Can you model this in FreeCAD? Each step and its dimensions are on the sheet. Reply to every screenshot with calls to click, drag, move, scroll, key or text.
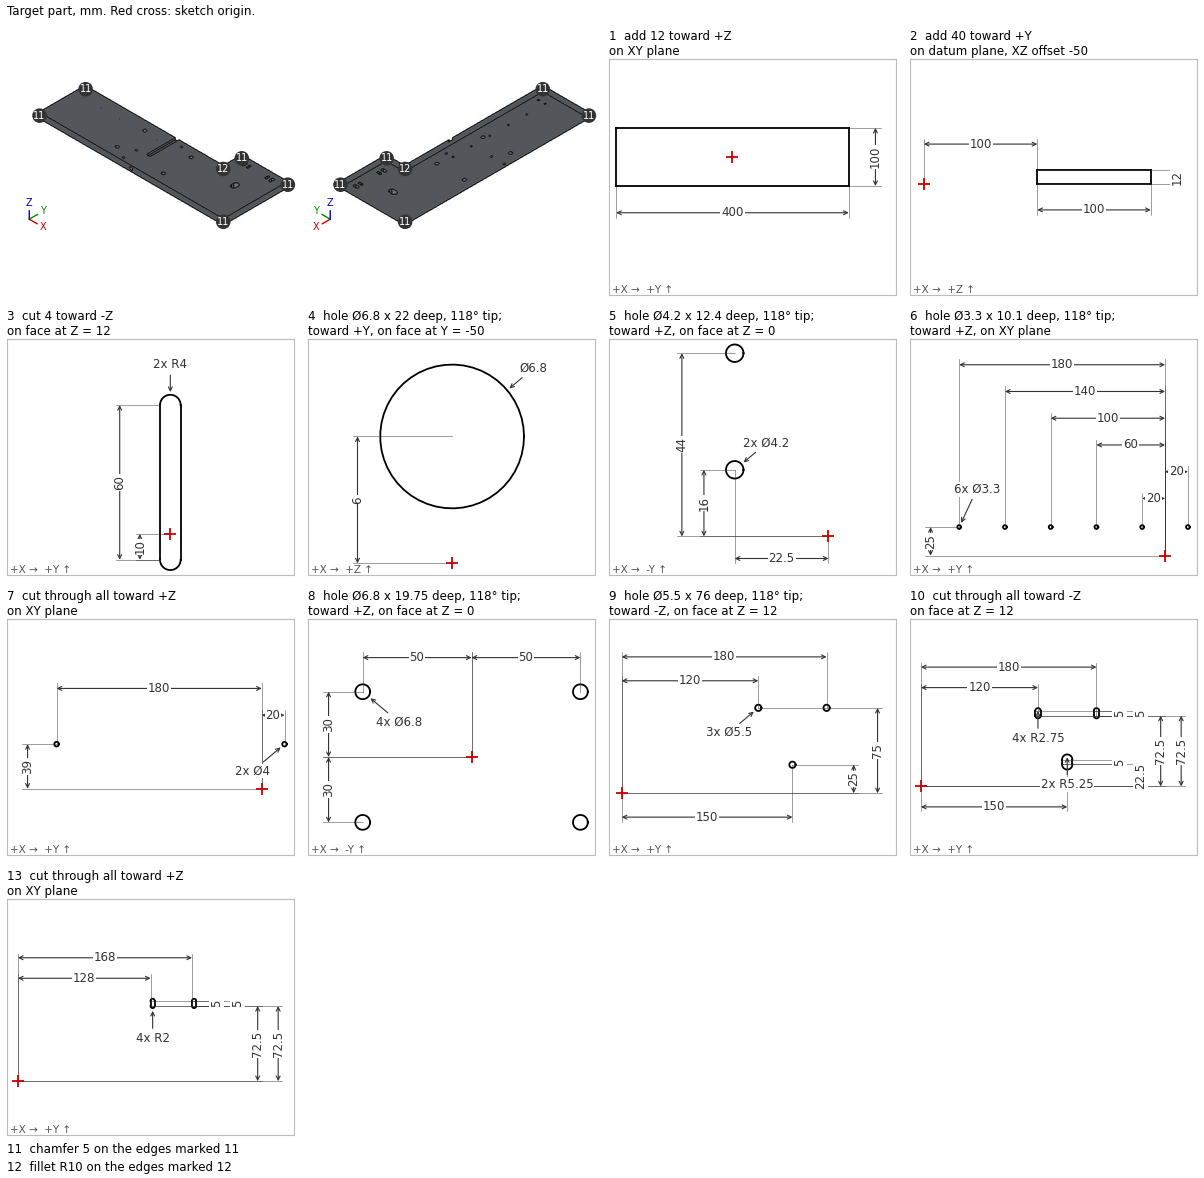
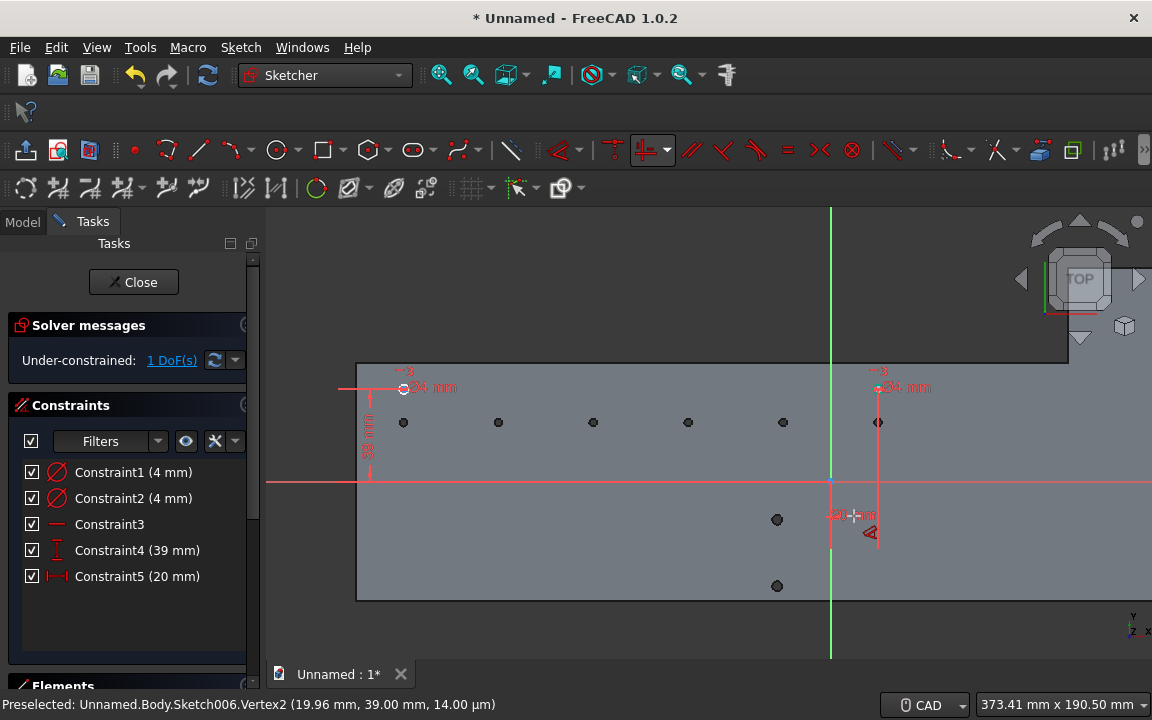
click(404, 389)
click(617, 516)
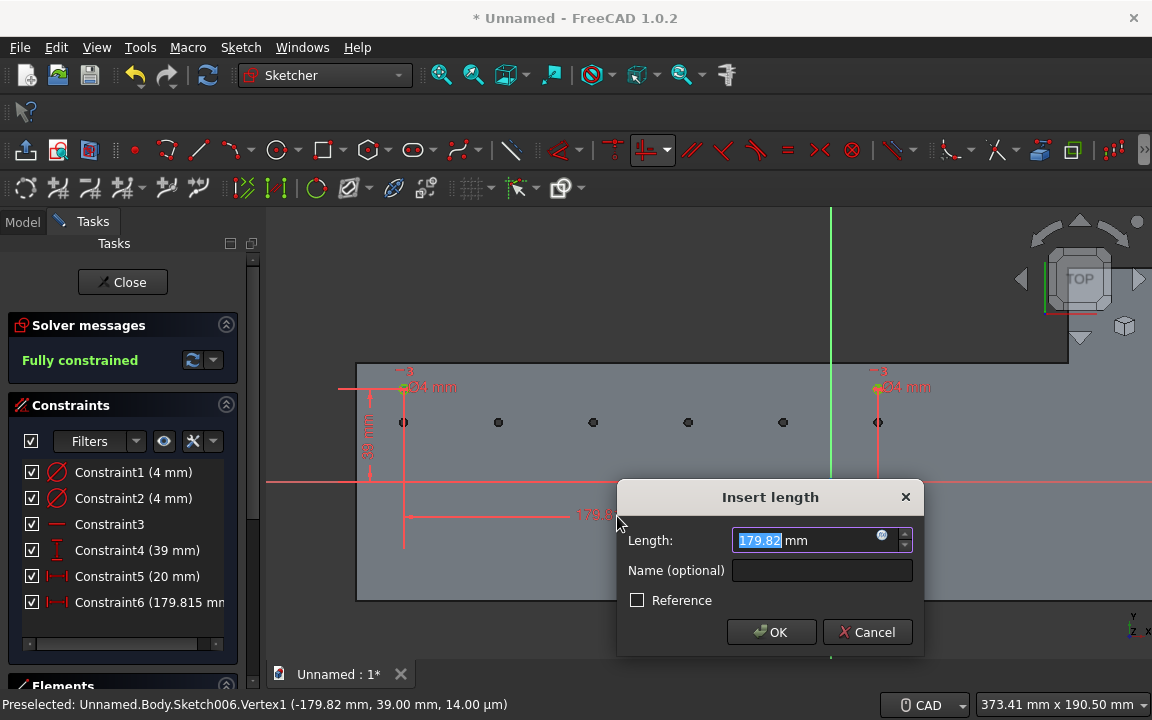
text(180)
key(Return)
key(Escape)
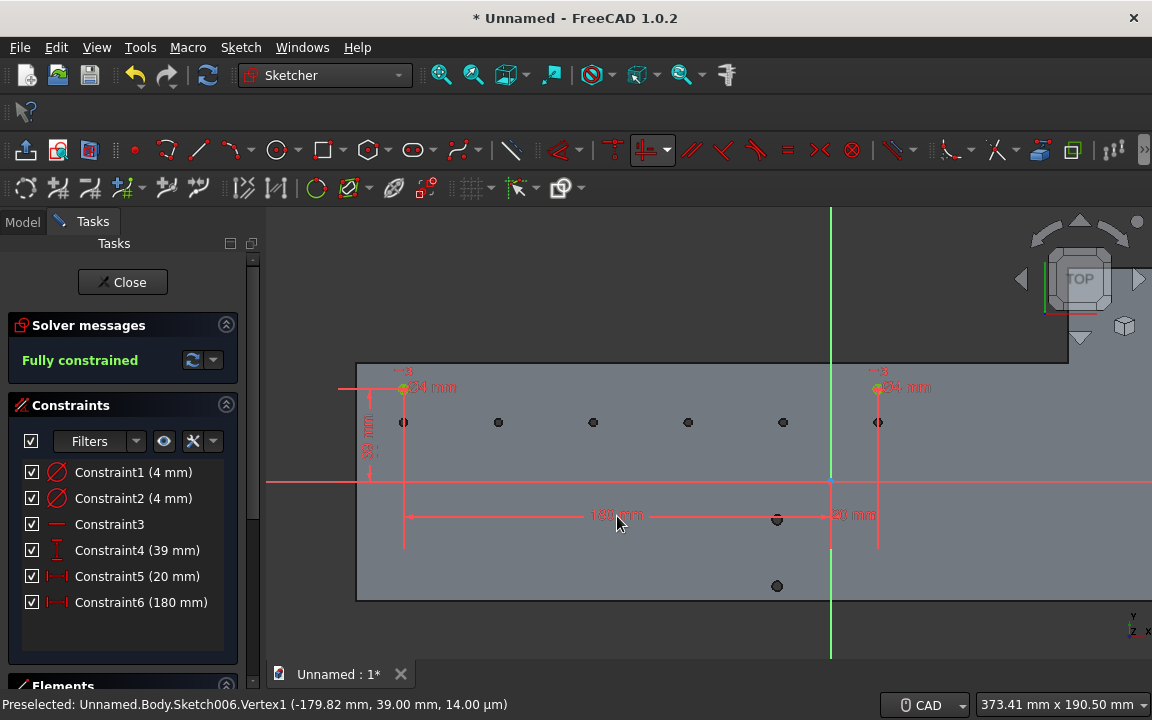
click(123, 282)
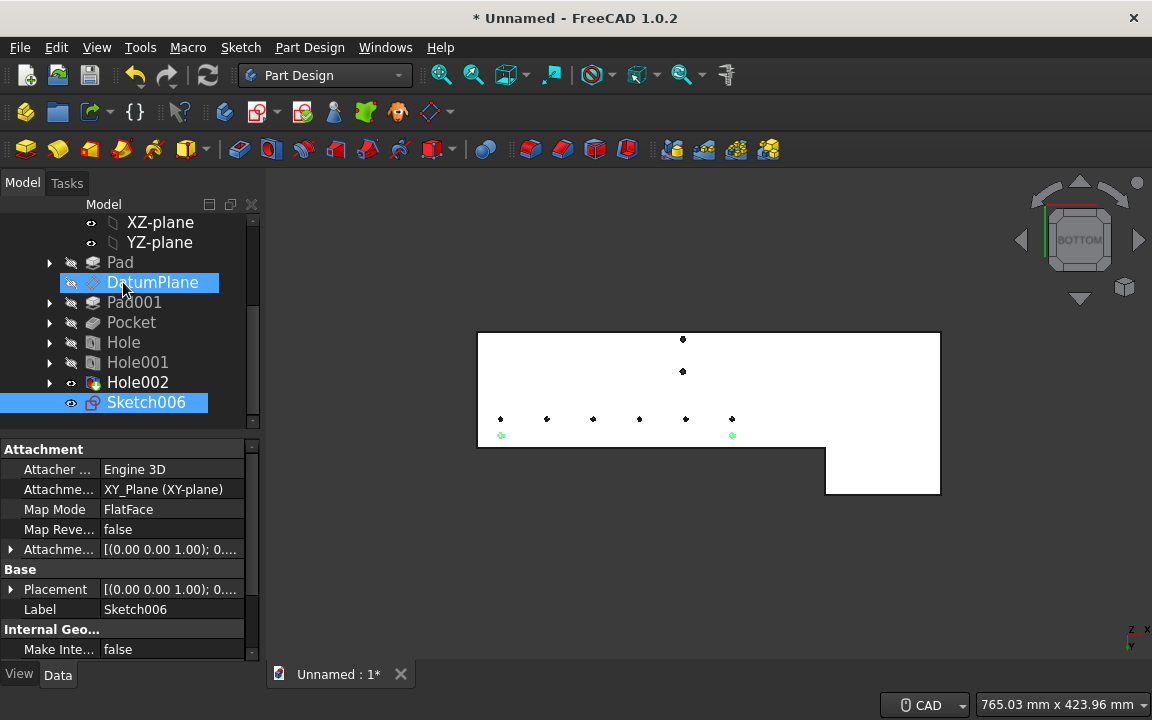
click(240, 150)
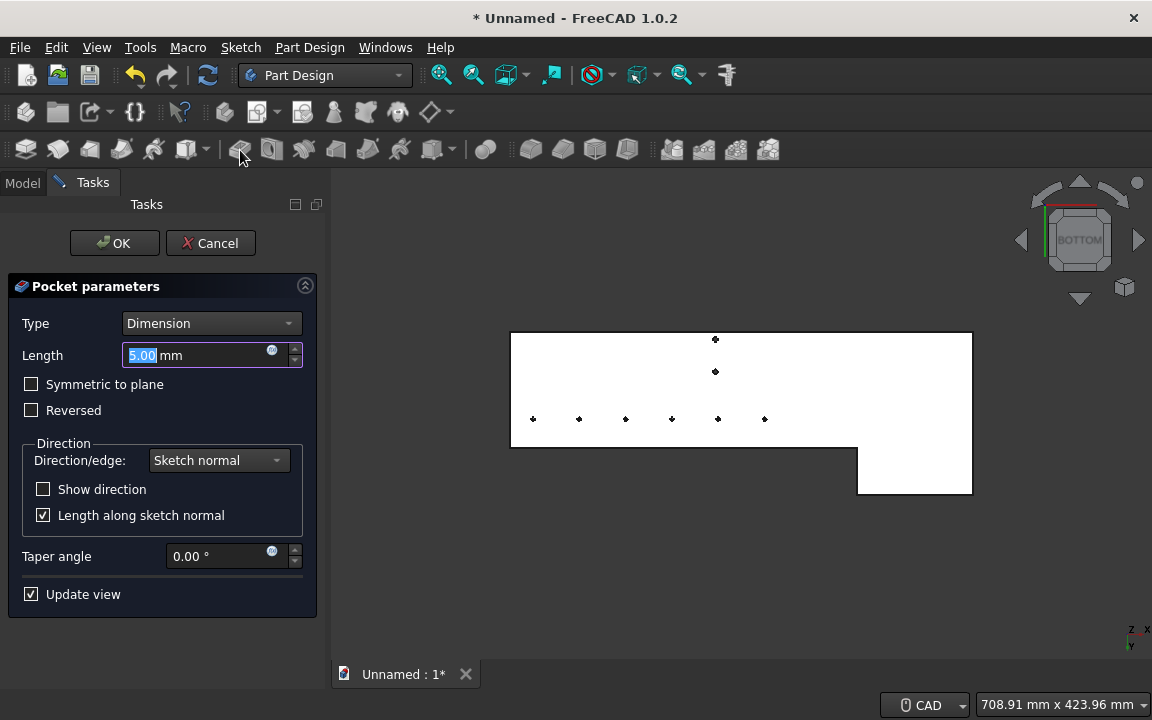
click(212, 324)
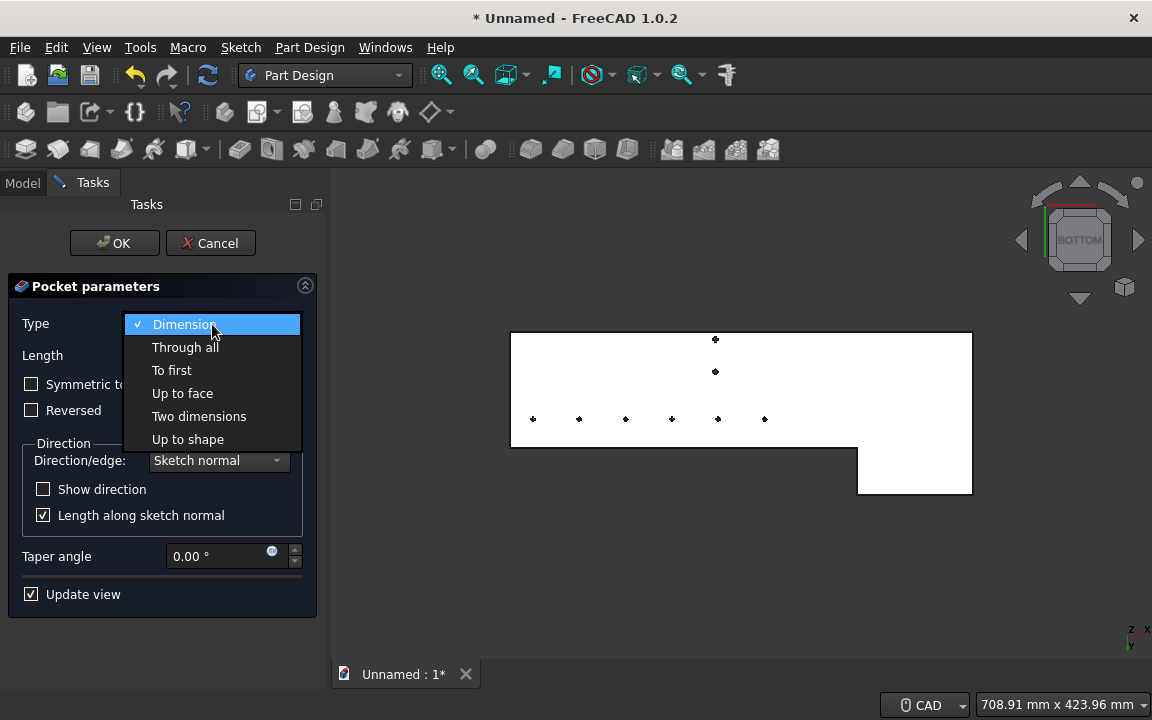
click(212, 348)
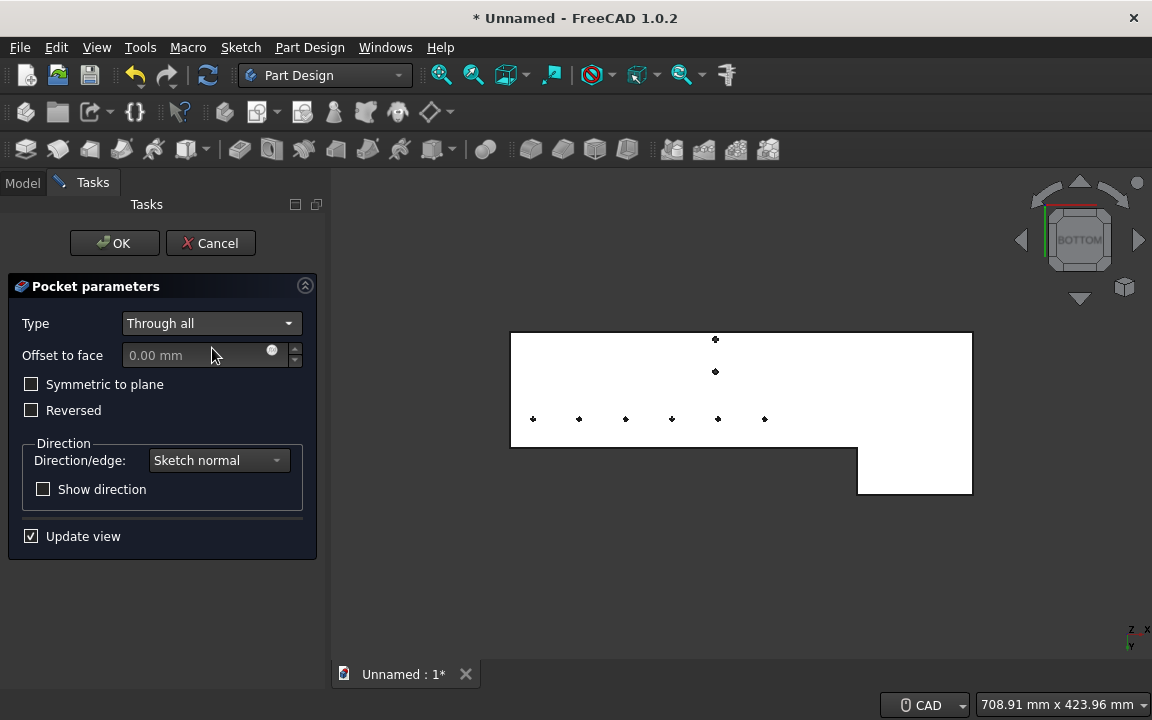
click(30, 410)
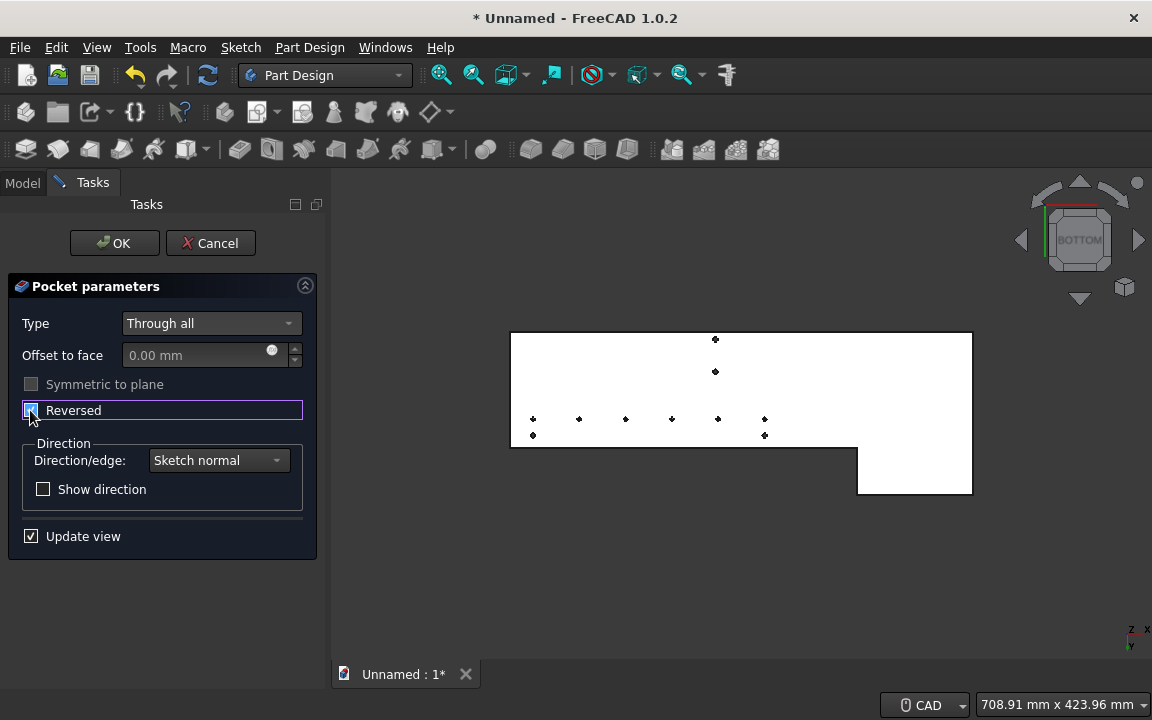
click(115, 243)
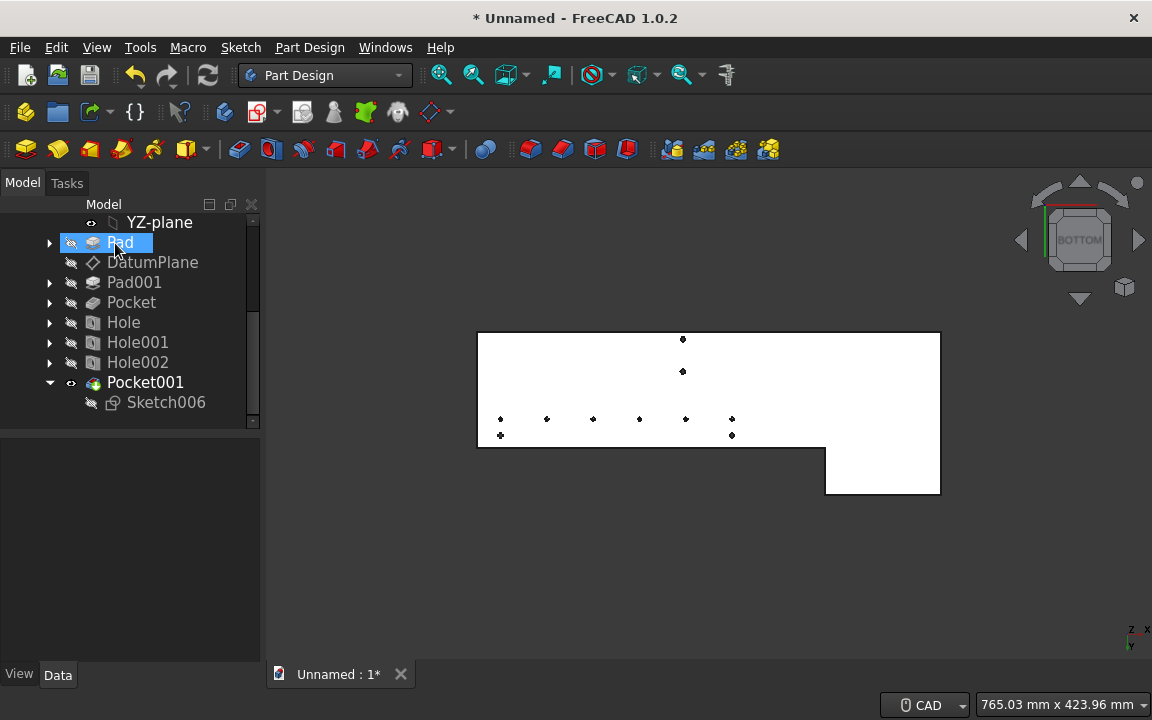
click(841, 389)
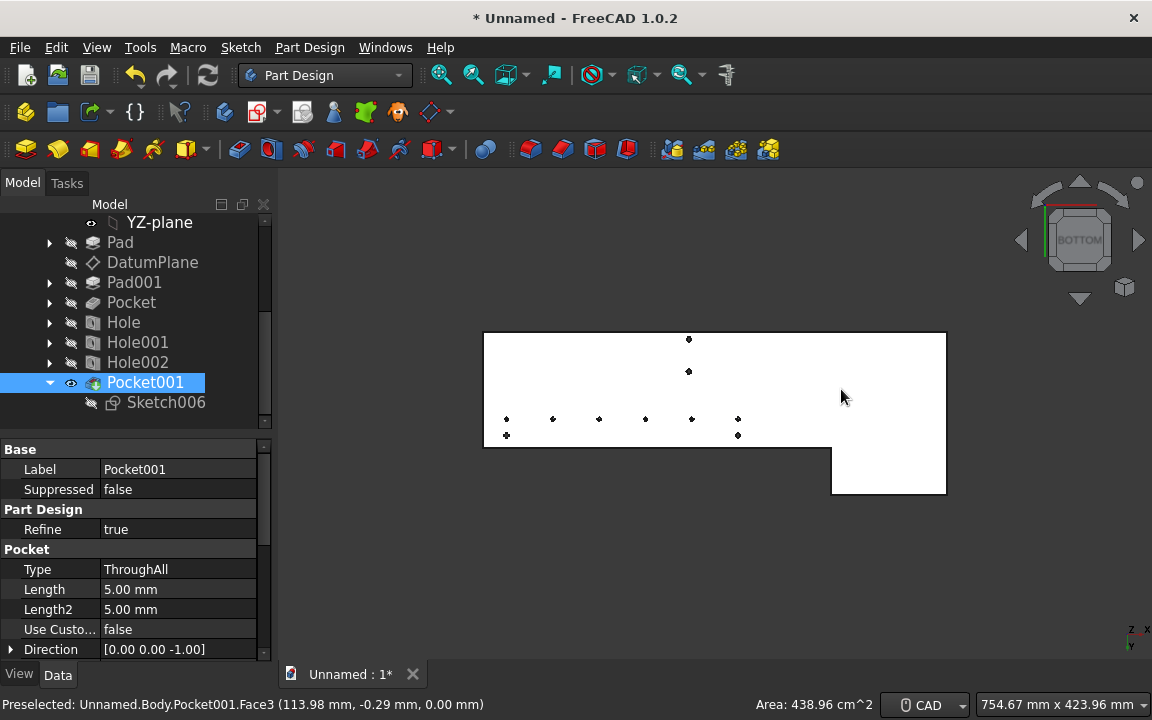
click(258, 112)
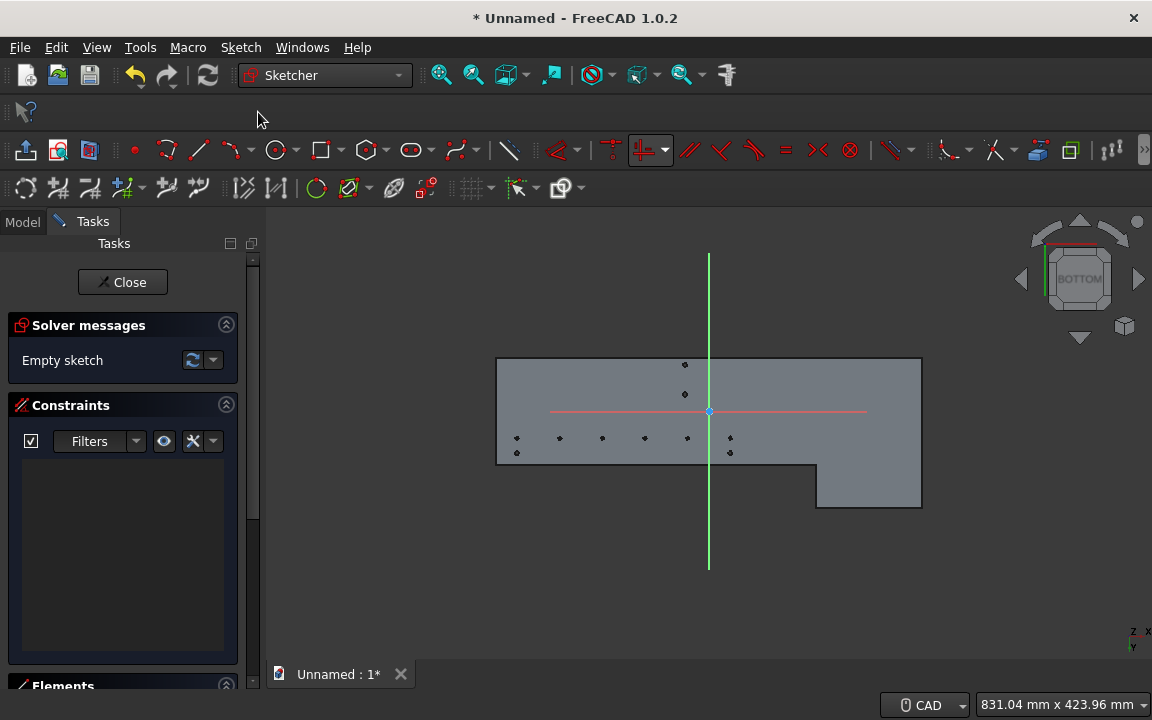
scroll(731, 405, up, 7)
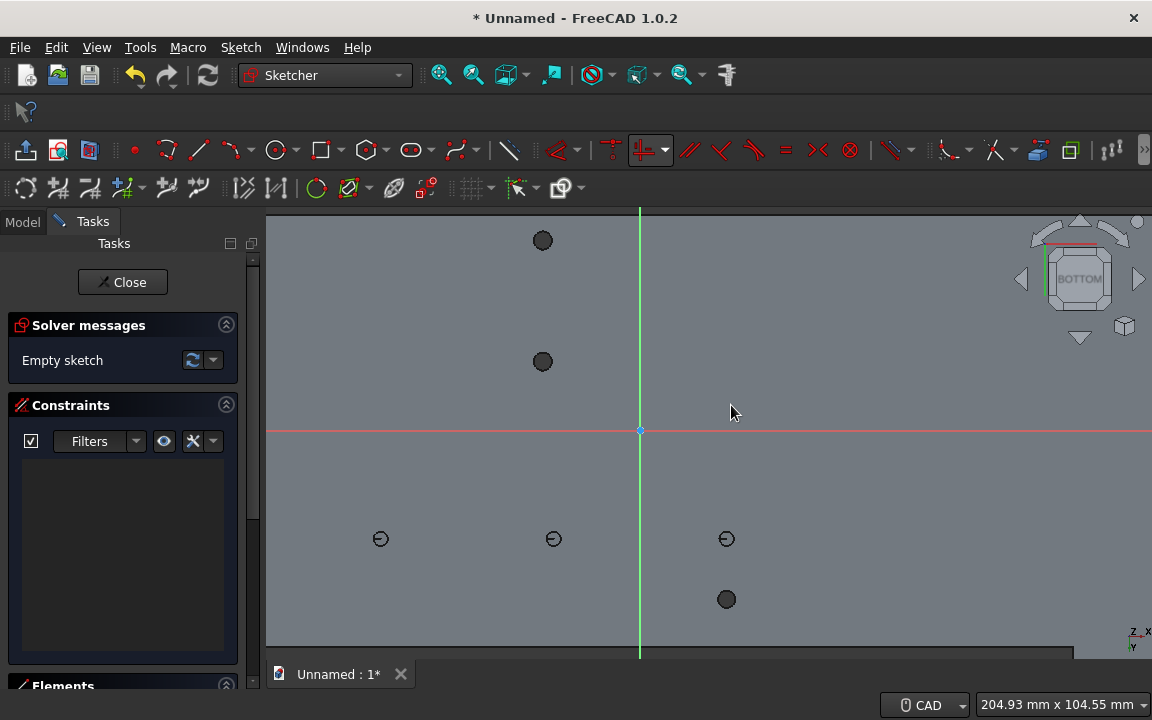
click(276, 150)